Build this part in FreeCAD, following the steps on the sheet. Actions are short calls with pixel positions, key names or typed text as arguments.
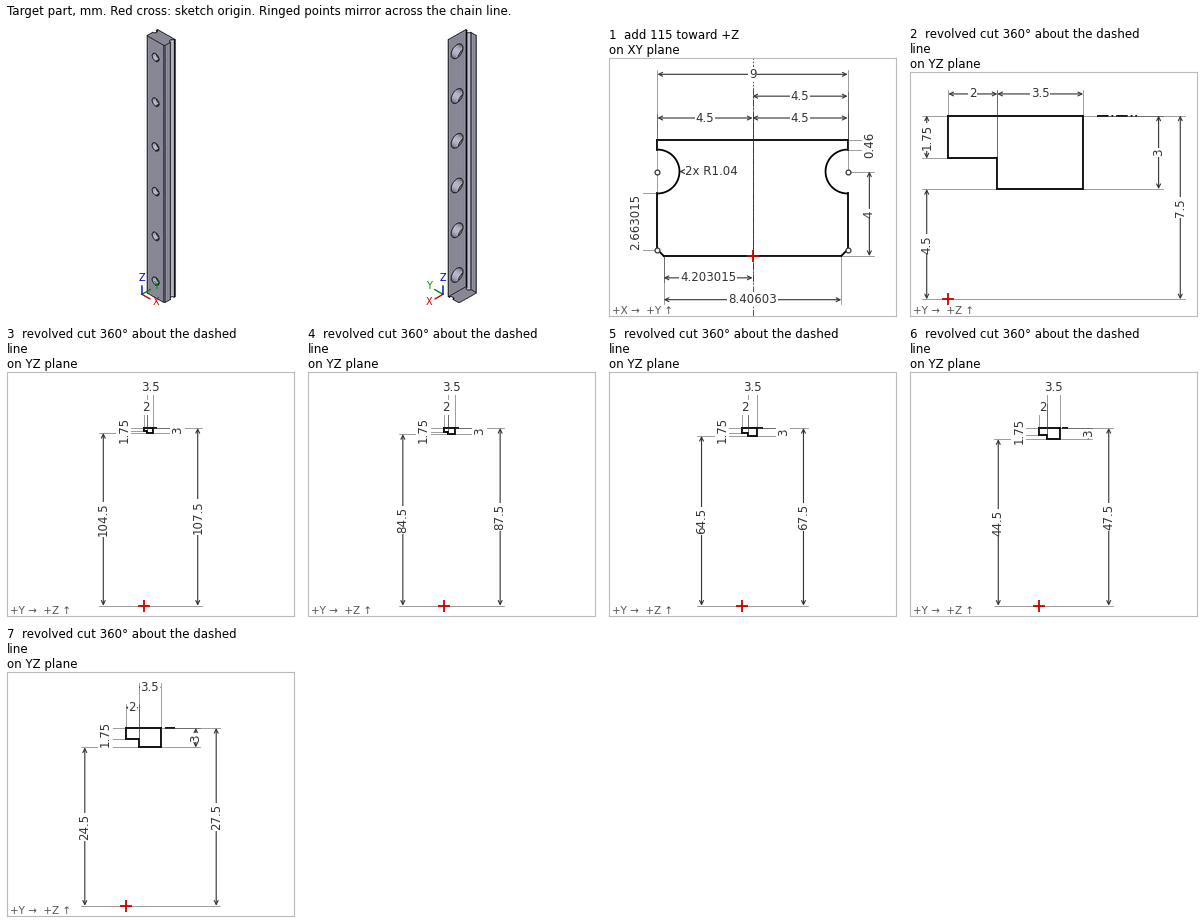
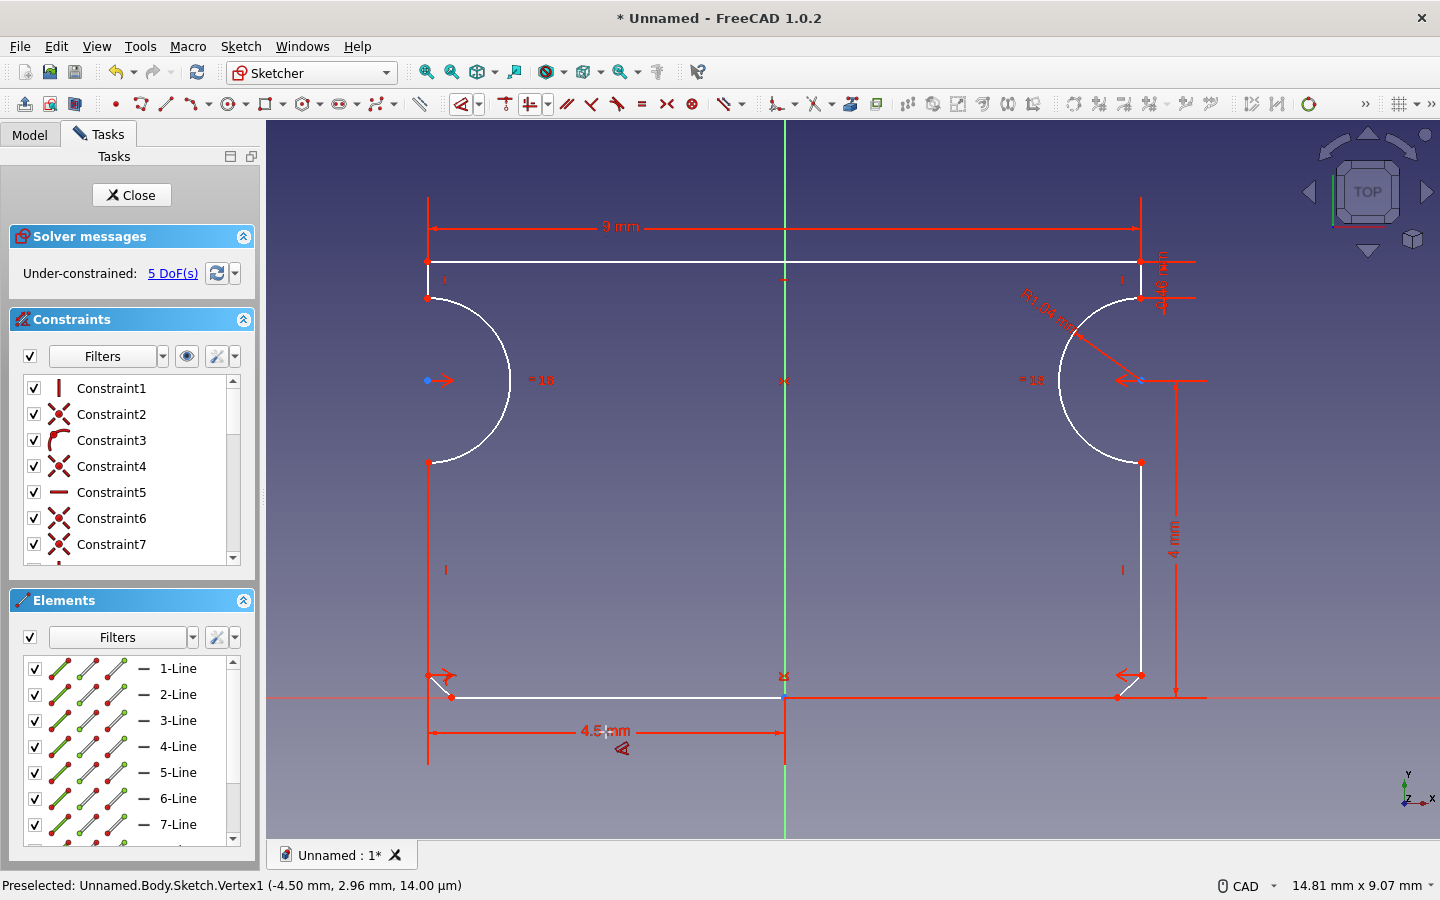
click(1141, 298)
click(963, 732)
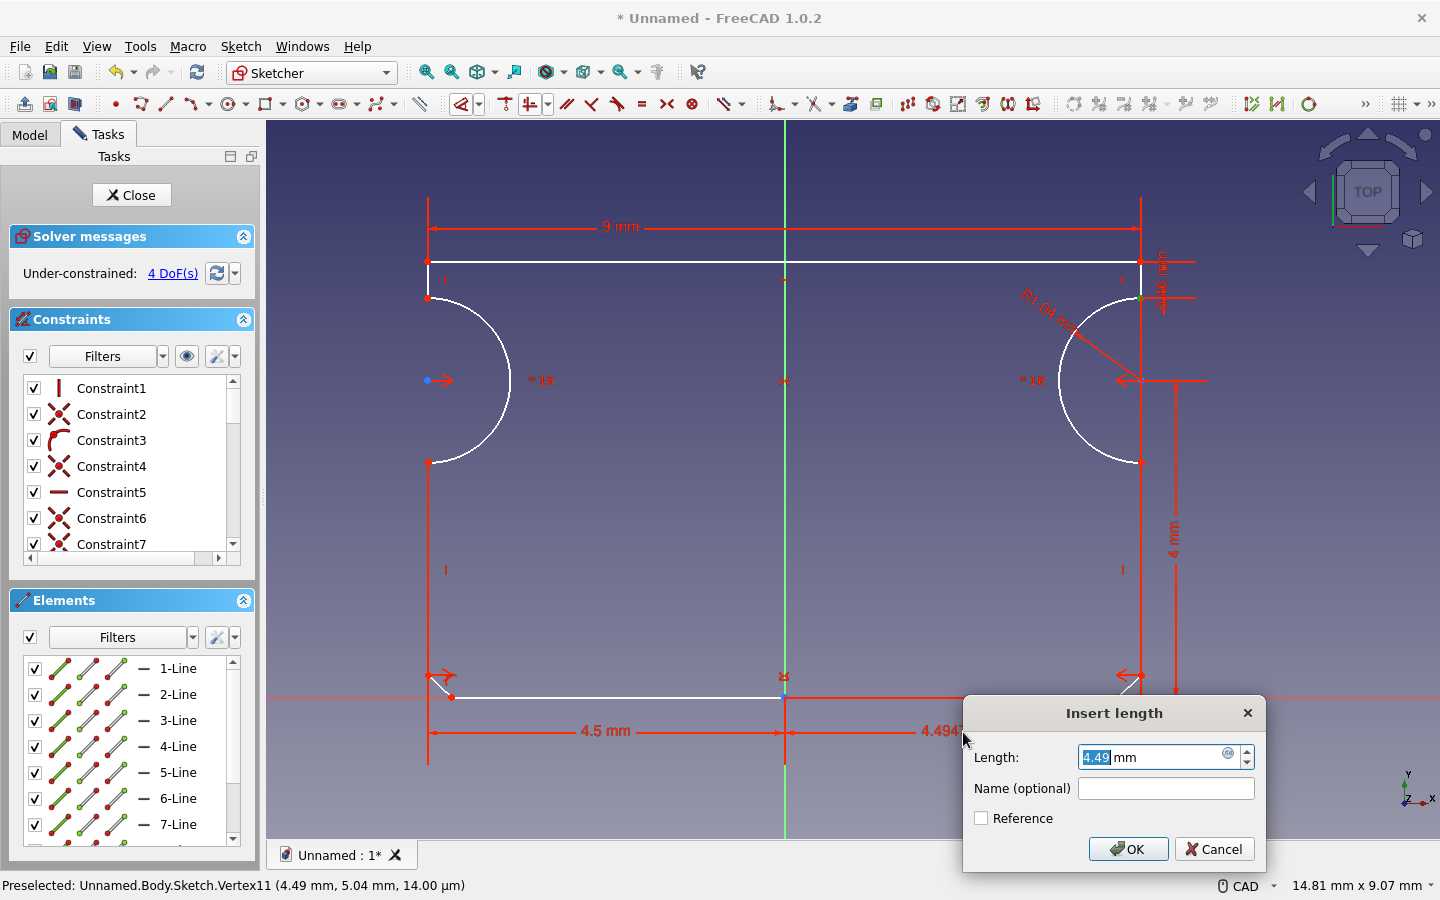
text(4.5)
key(Return)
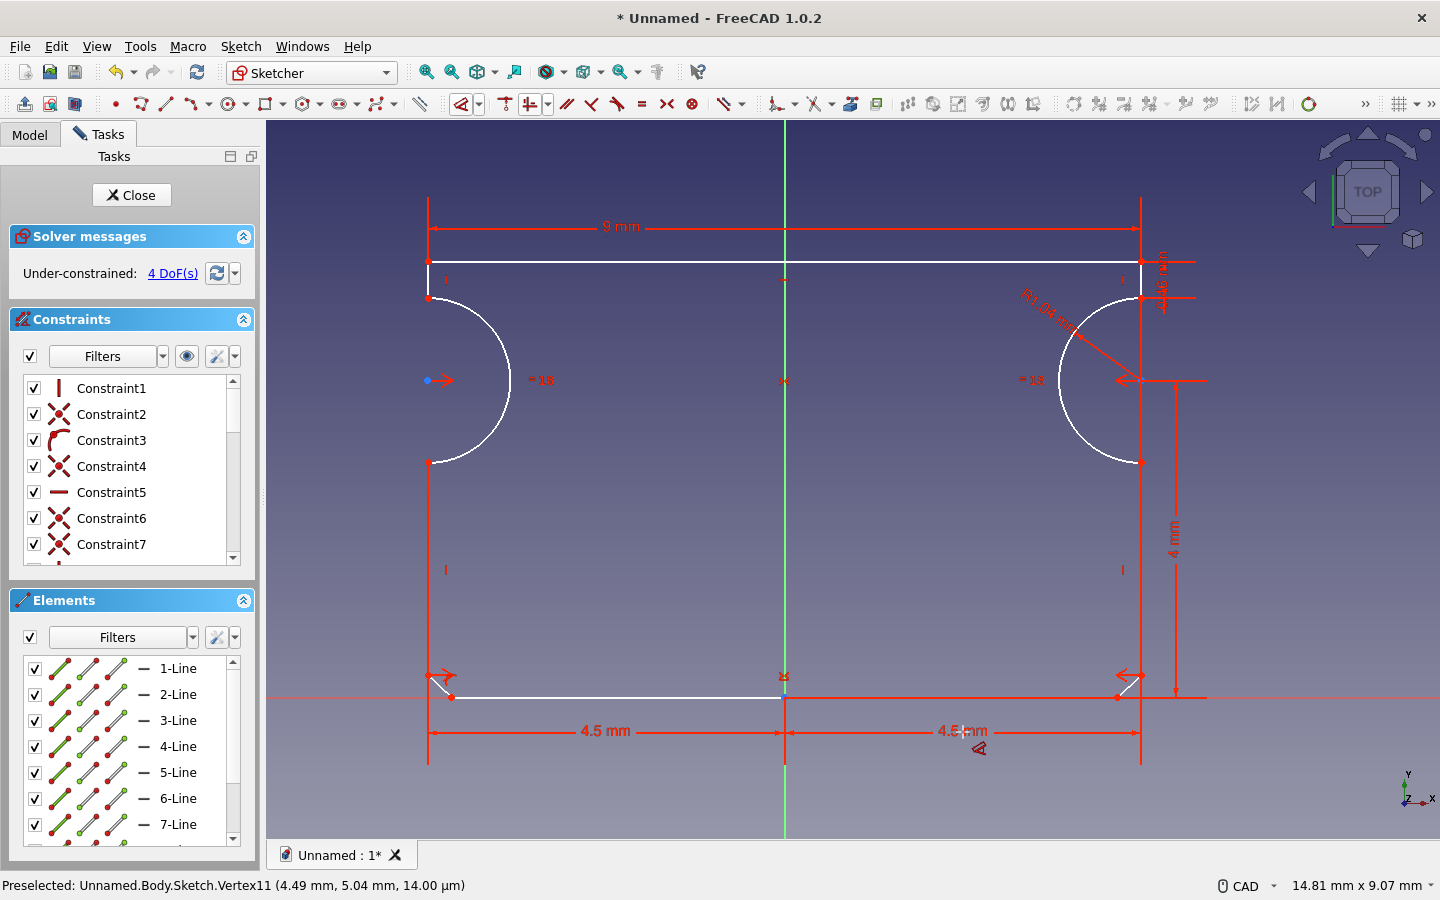
click(1141, 381)
click(881, 732)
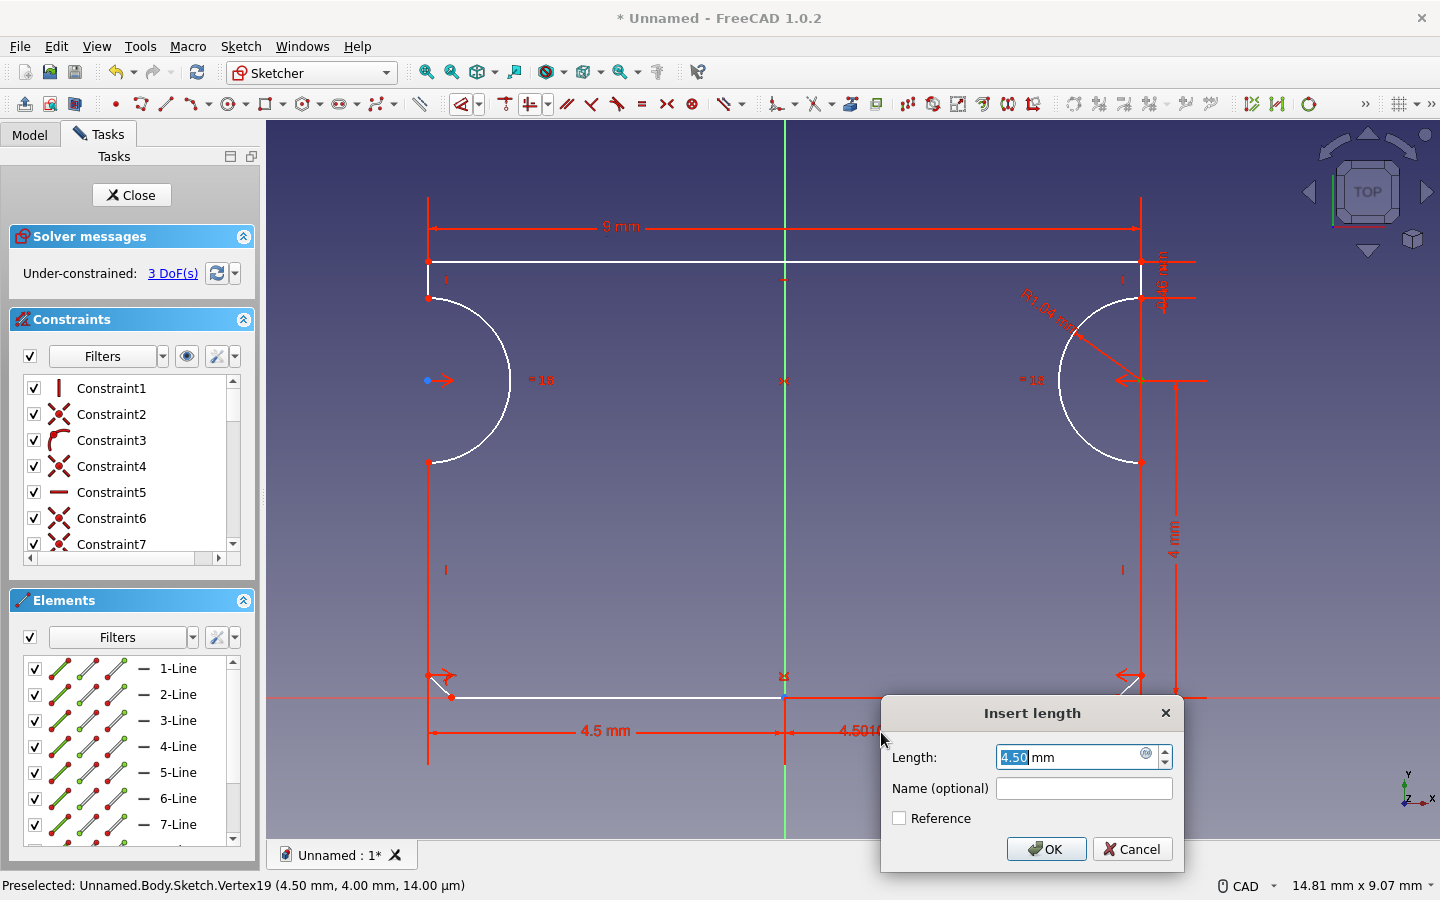
text(4.5)
key(Return)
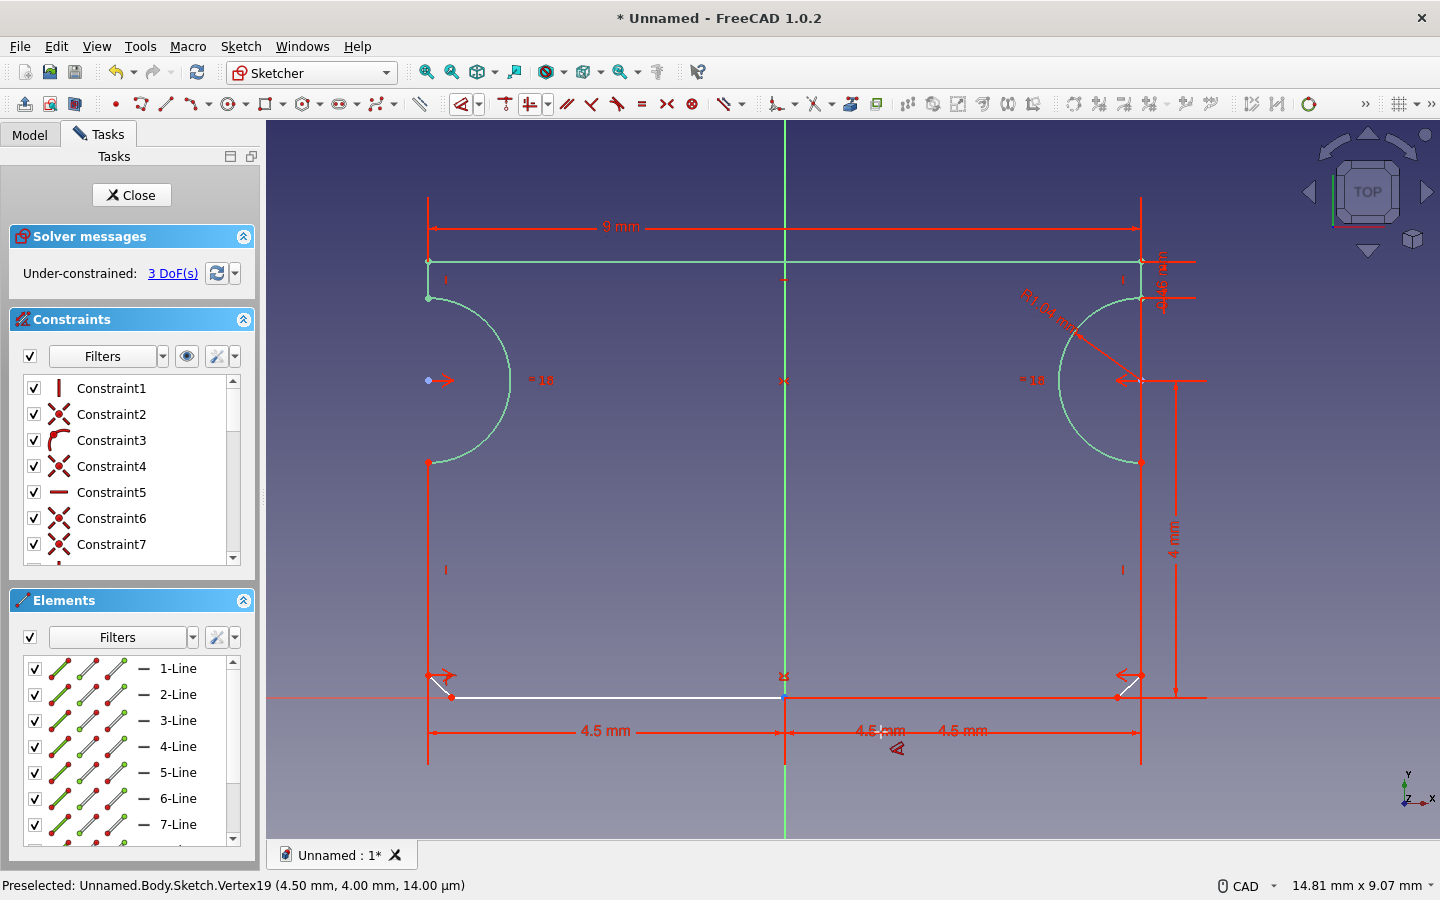
click(652, 698)
click(632, 664)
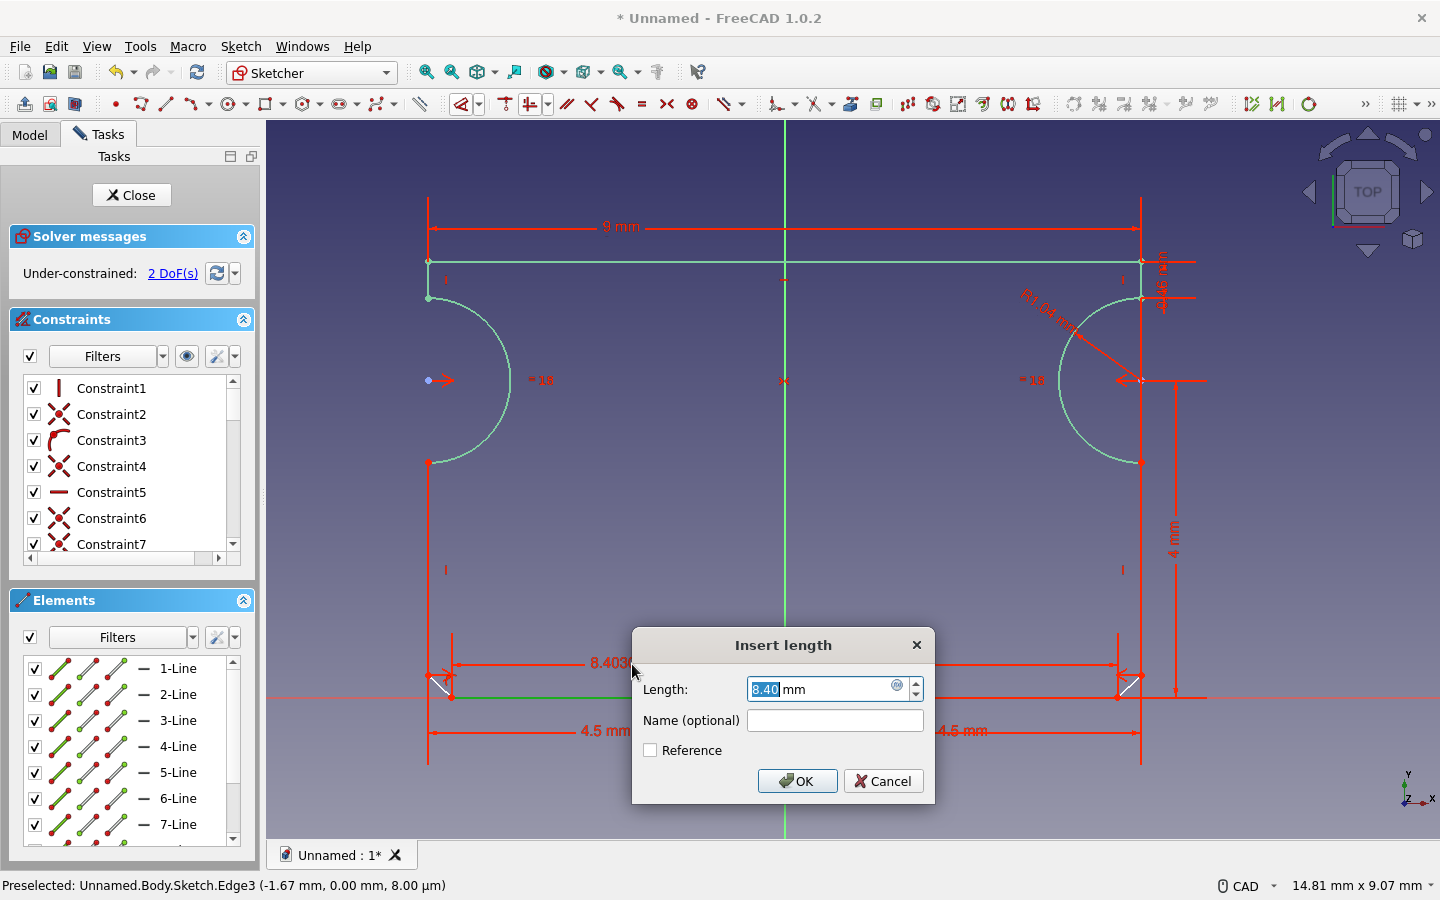
text(8.40603)
key(Return)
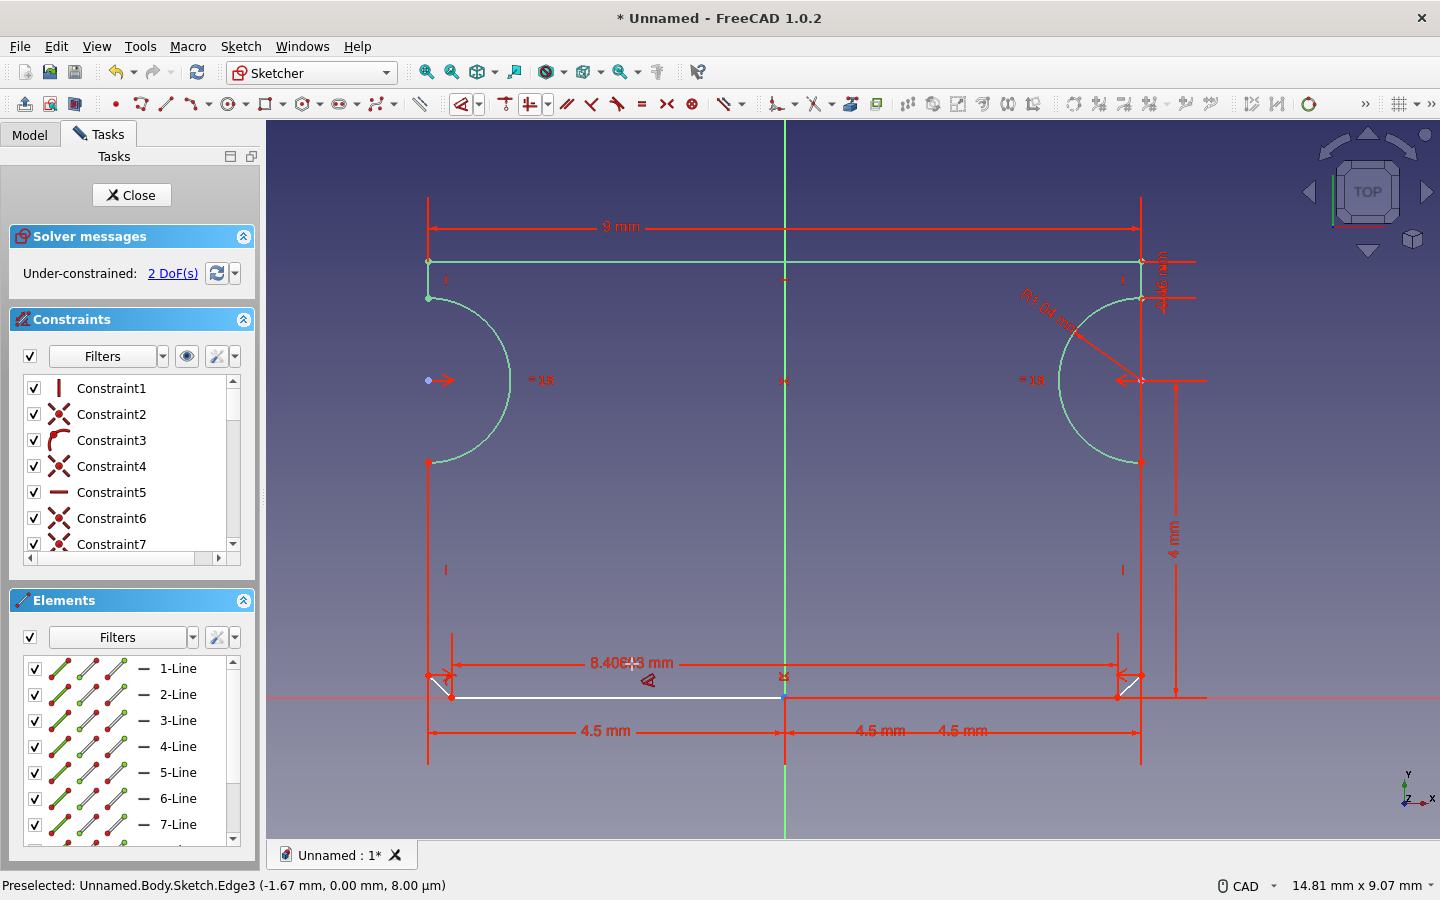
click(428, 527)
click(394, 569)